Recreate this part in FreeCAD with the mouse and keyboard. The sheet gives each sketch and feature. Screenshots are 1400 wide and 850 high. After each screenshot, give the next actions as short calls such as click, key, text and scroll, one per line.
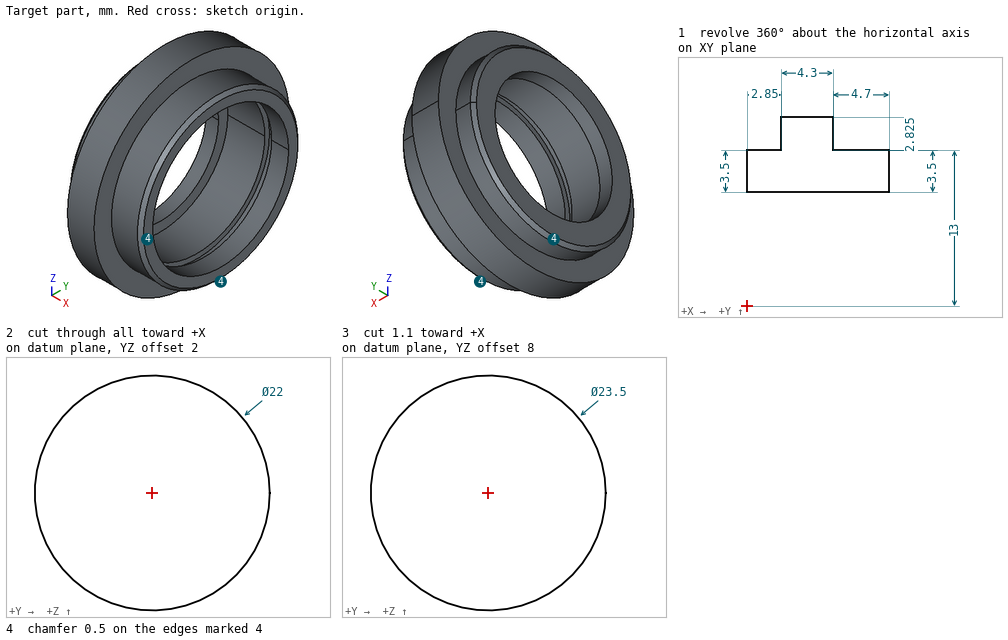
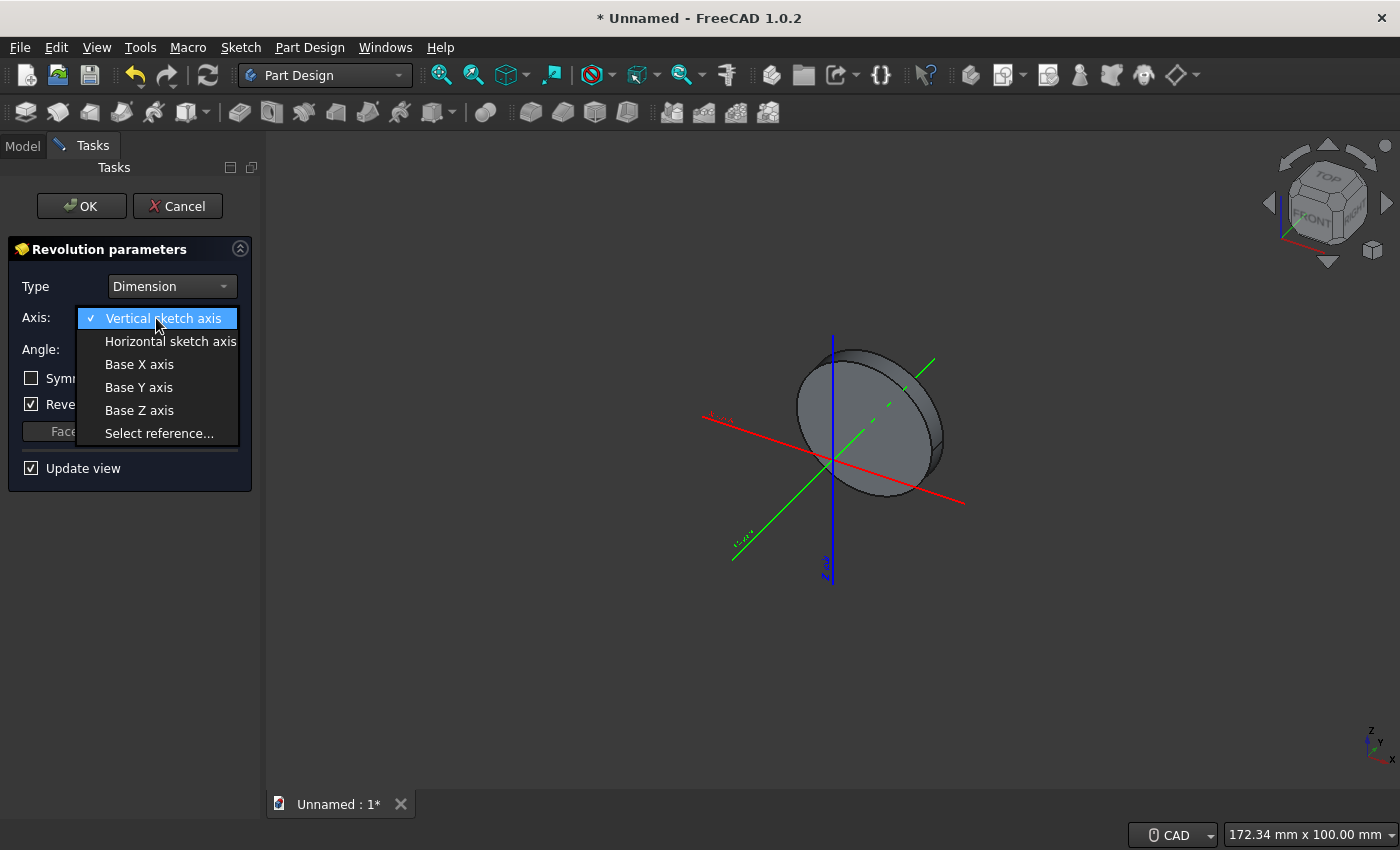
click(156, 342)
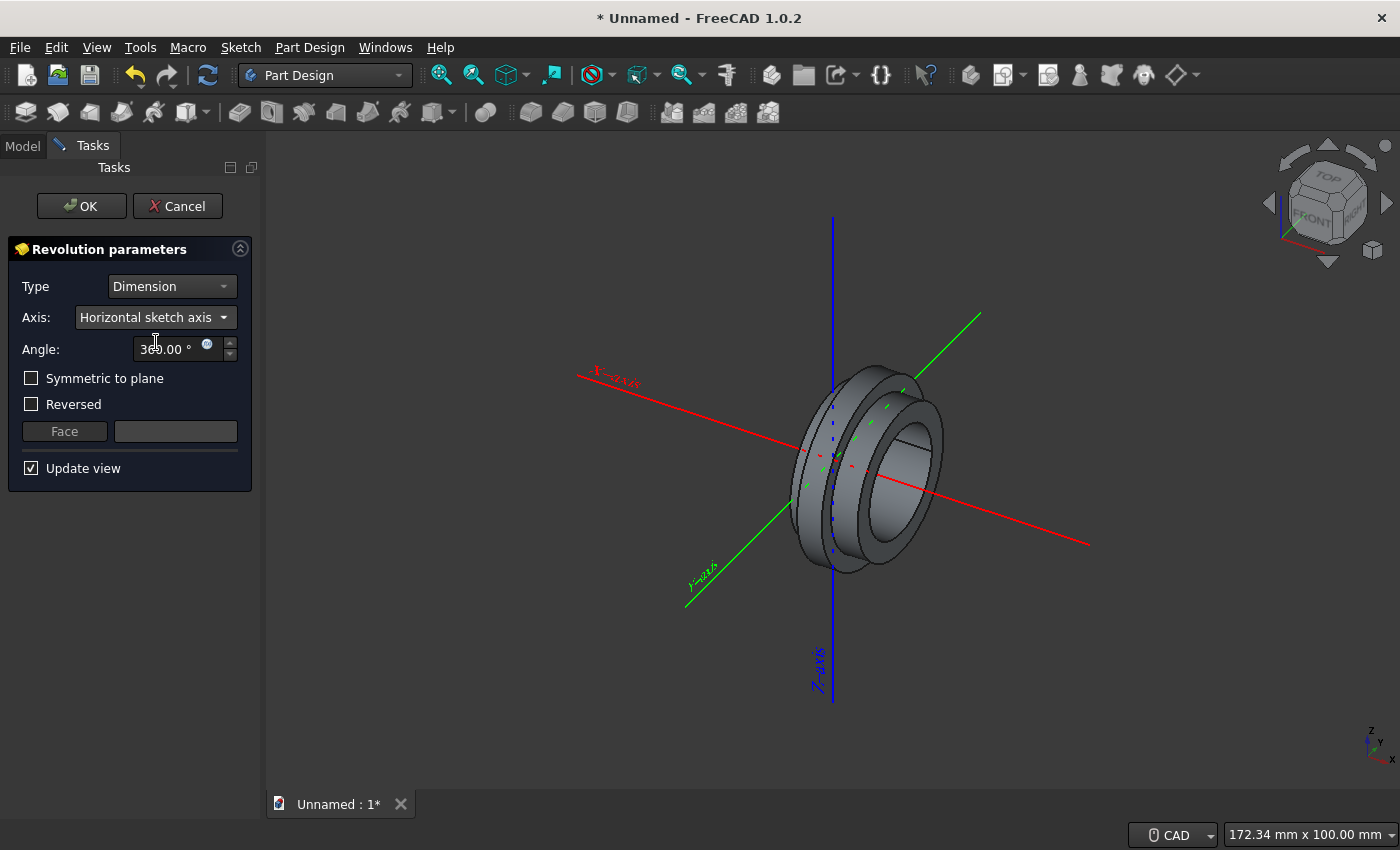
click(82, 206)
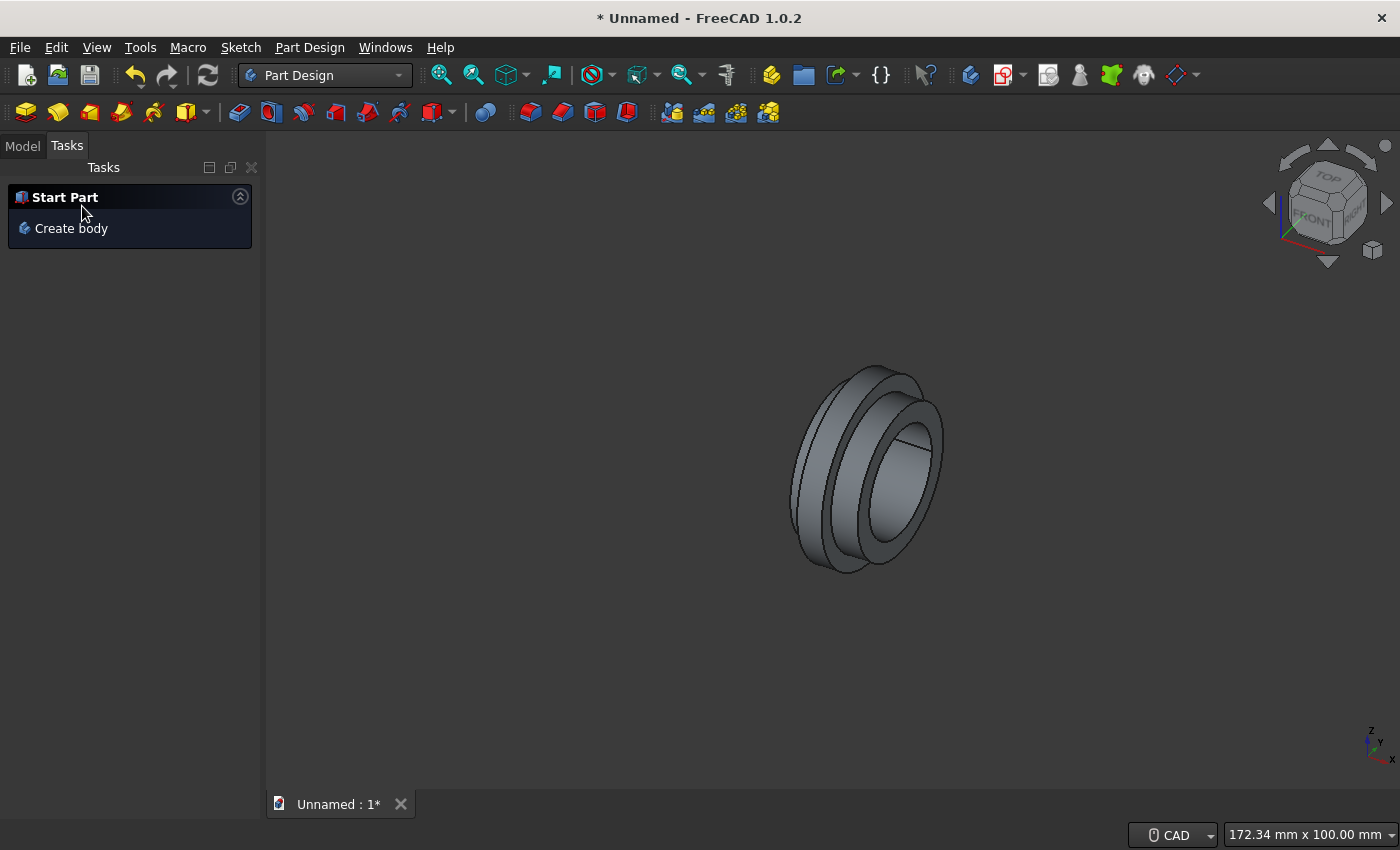
click(442, 76)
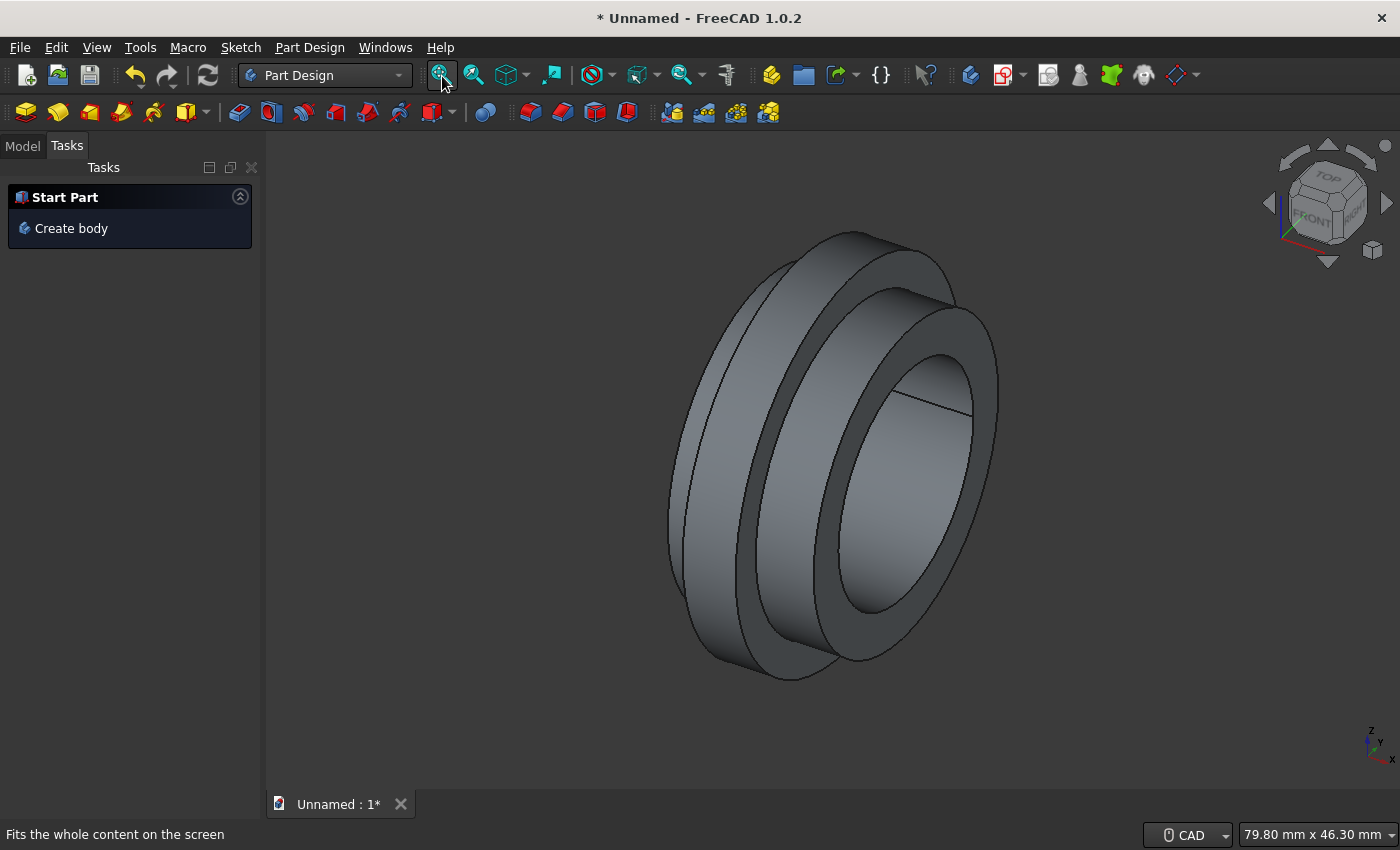
click(23, 145)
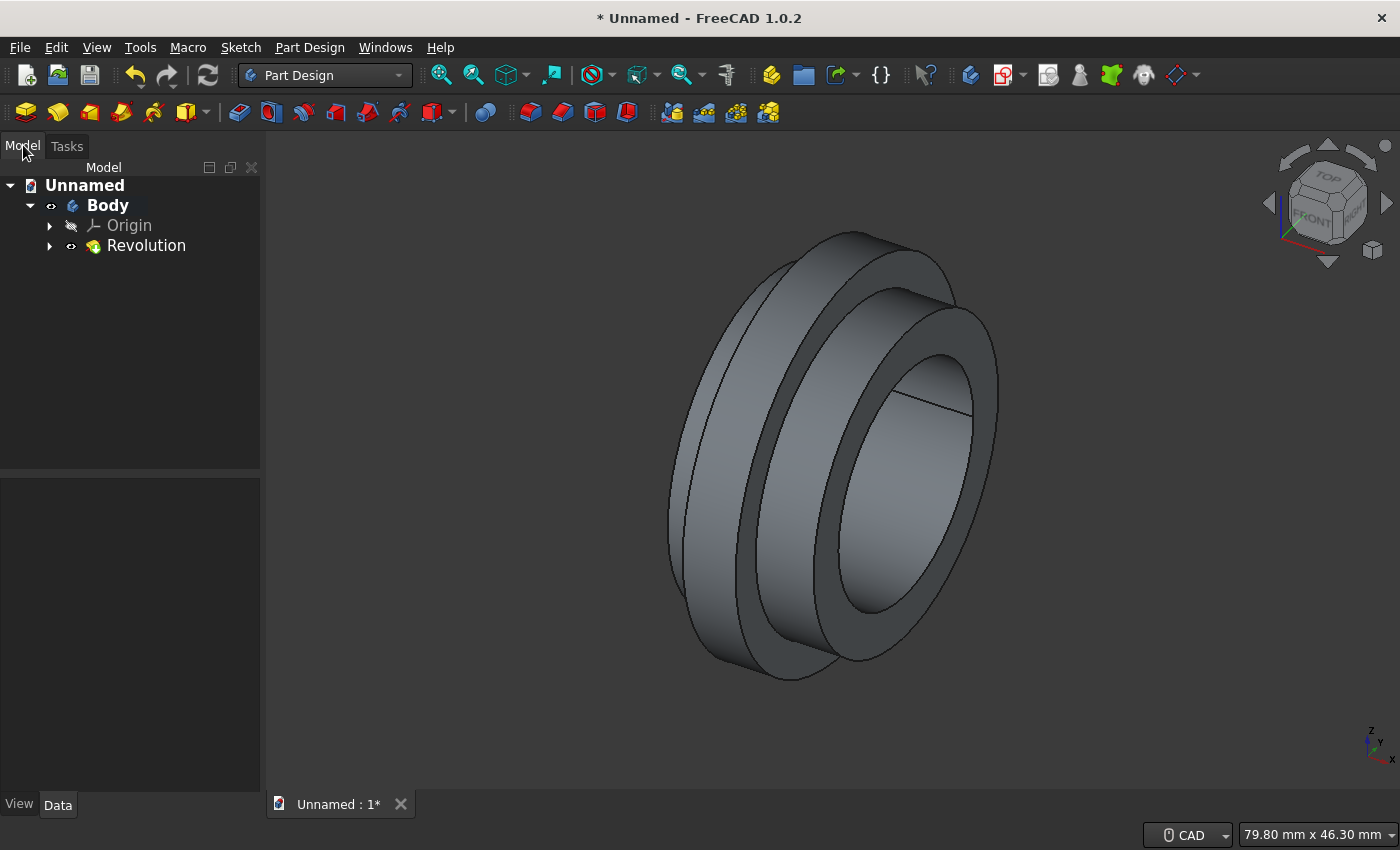
click(50, 226)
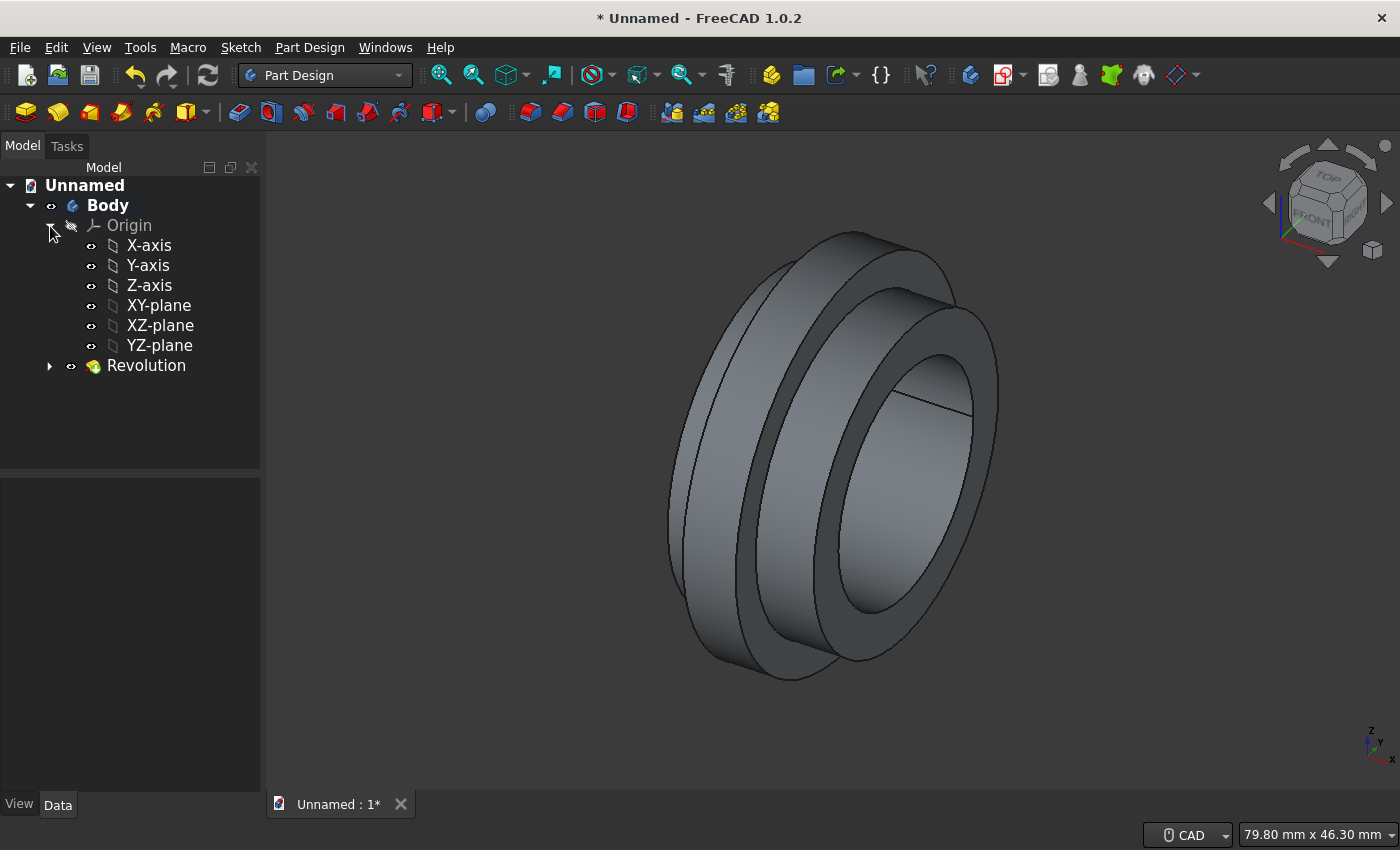
click(136, 346)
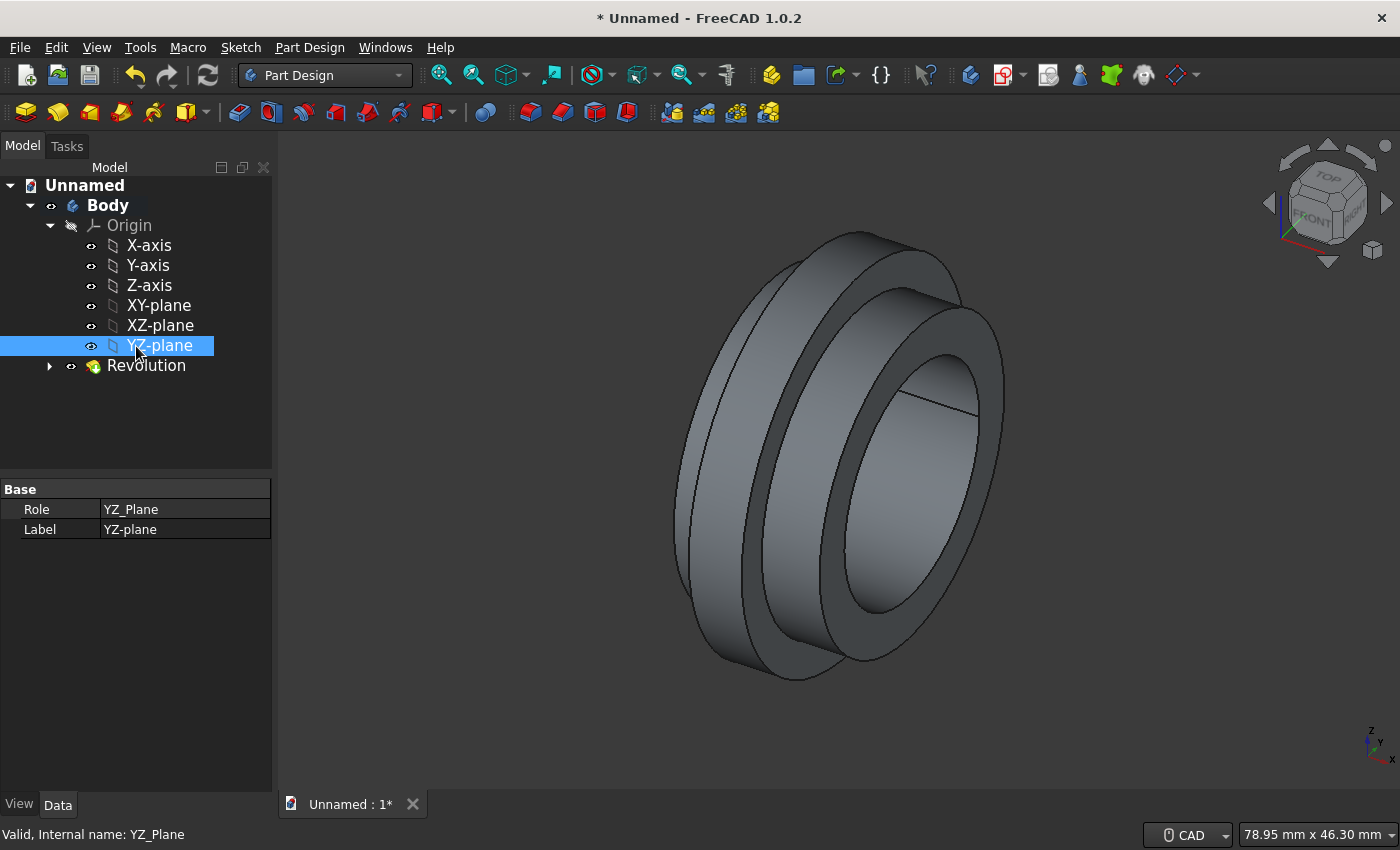
click(1176, 76)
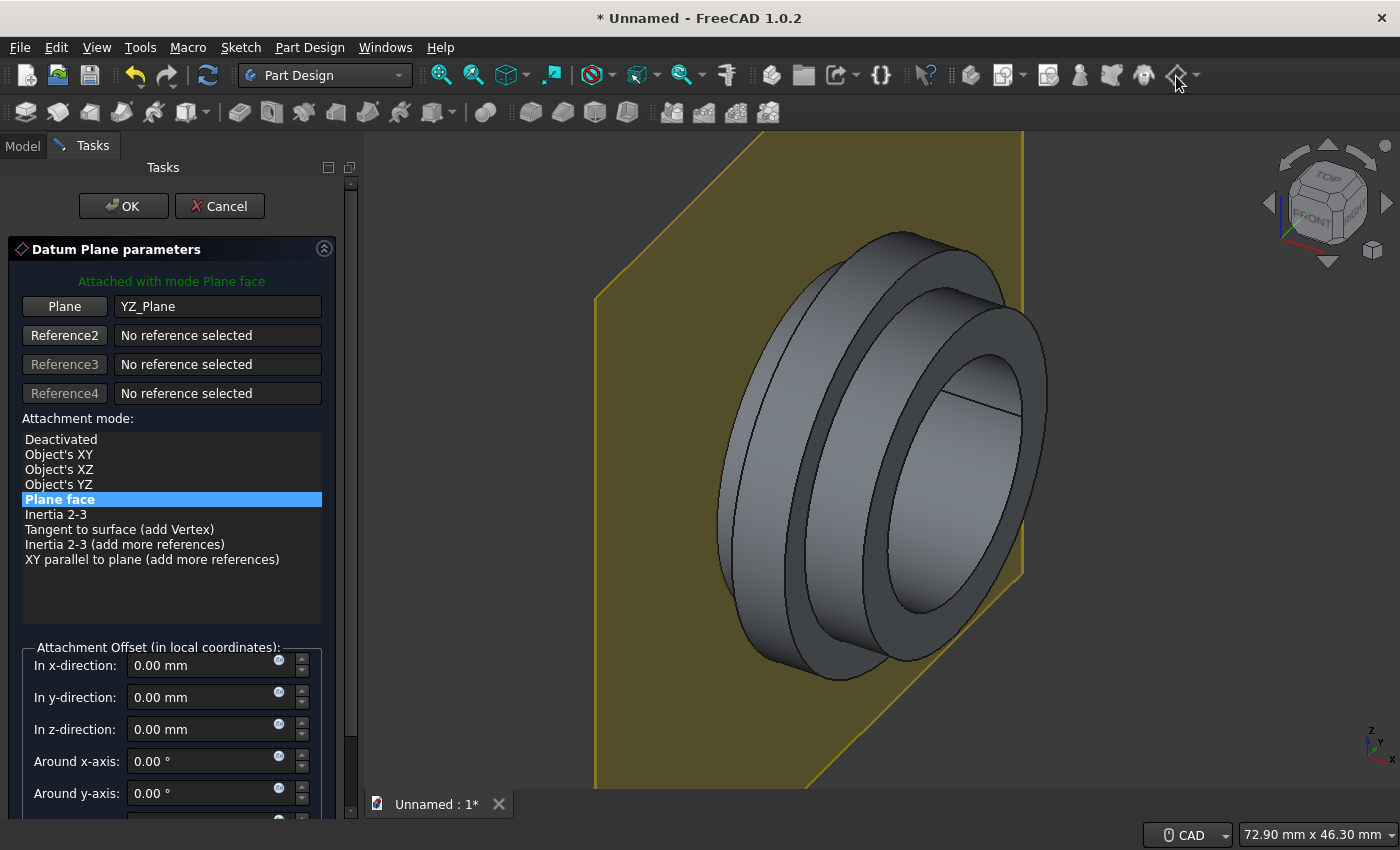
triple_click(210, 729)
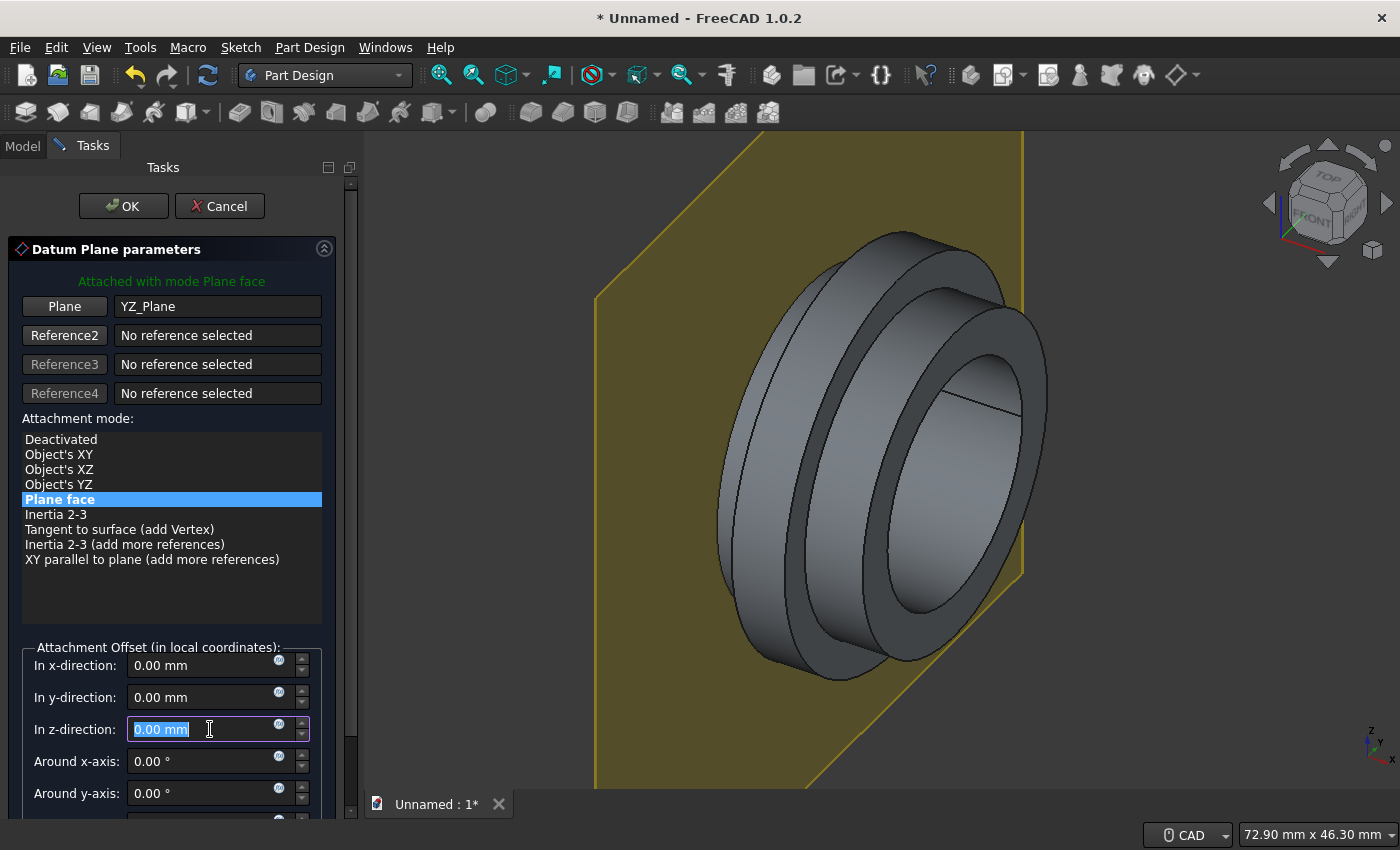
text(2)
key(Tab)